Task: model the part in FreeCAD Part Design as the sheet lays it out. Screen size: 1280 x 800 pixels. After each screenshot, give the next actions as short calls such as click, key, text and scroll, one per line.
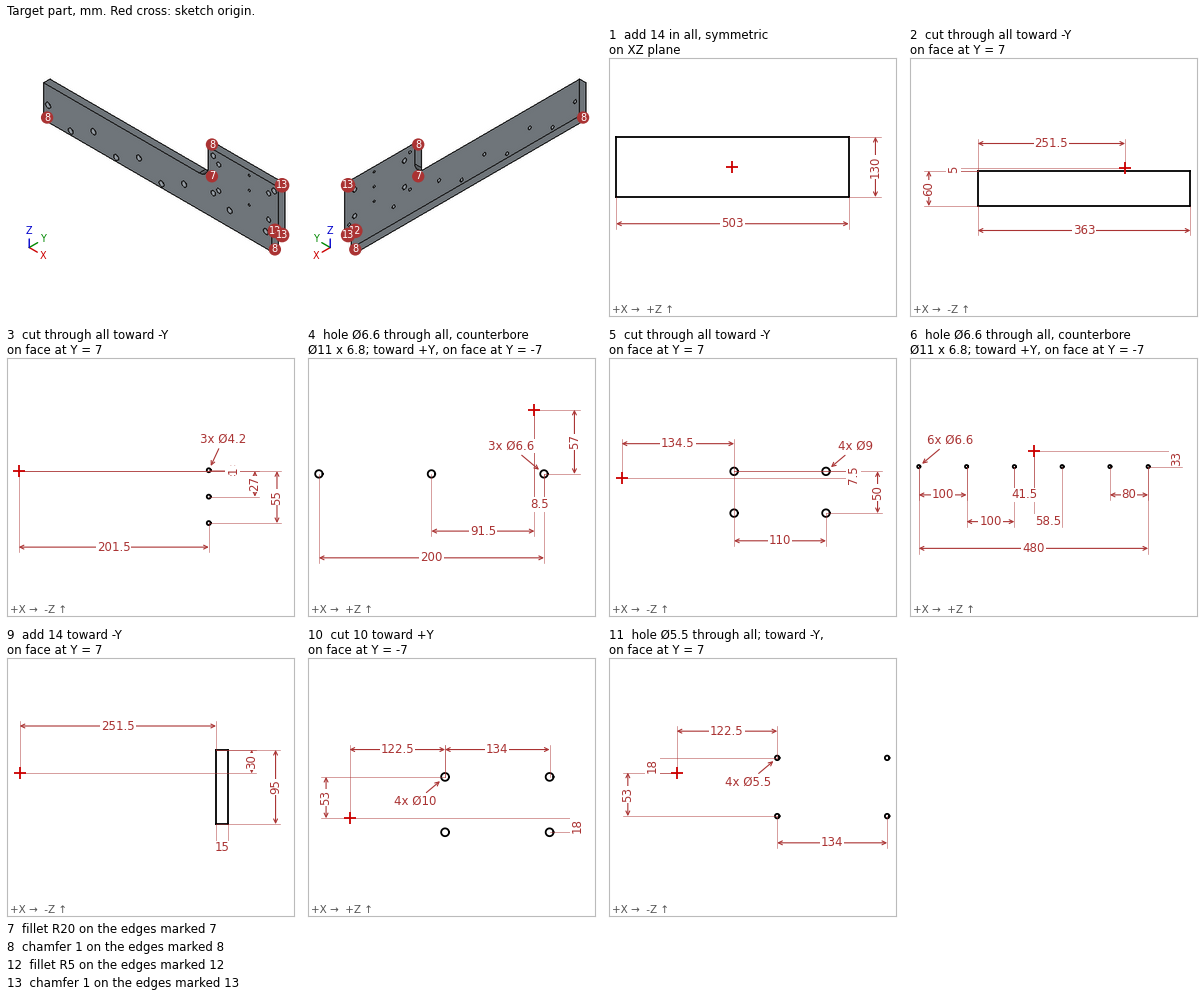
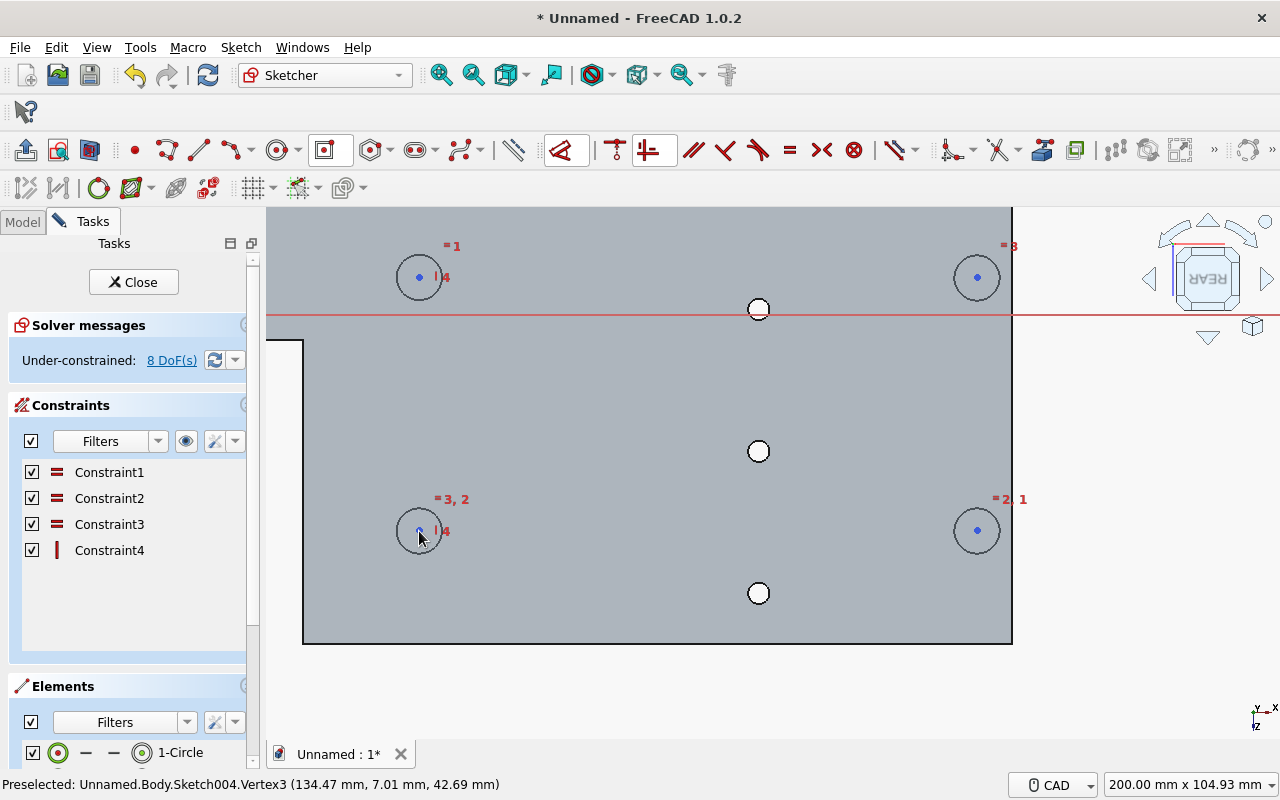
click(977, 531)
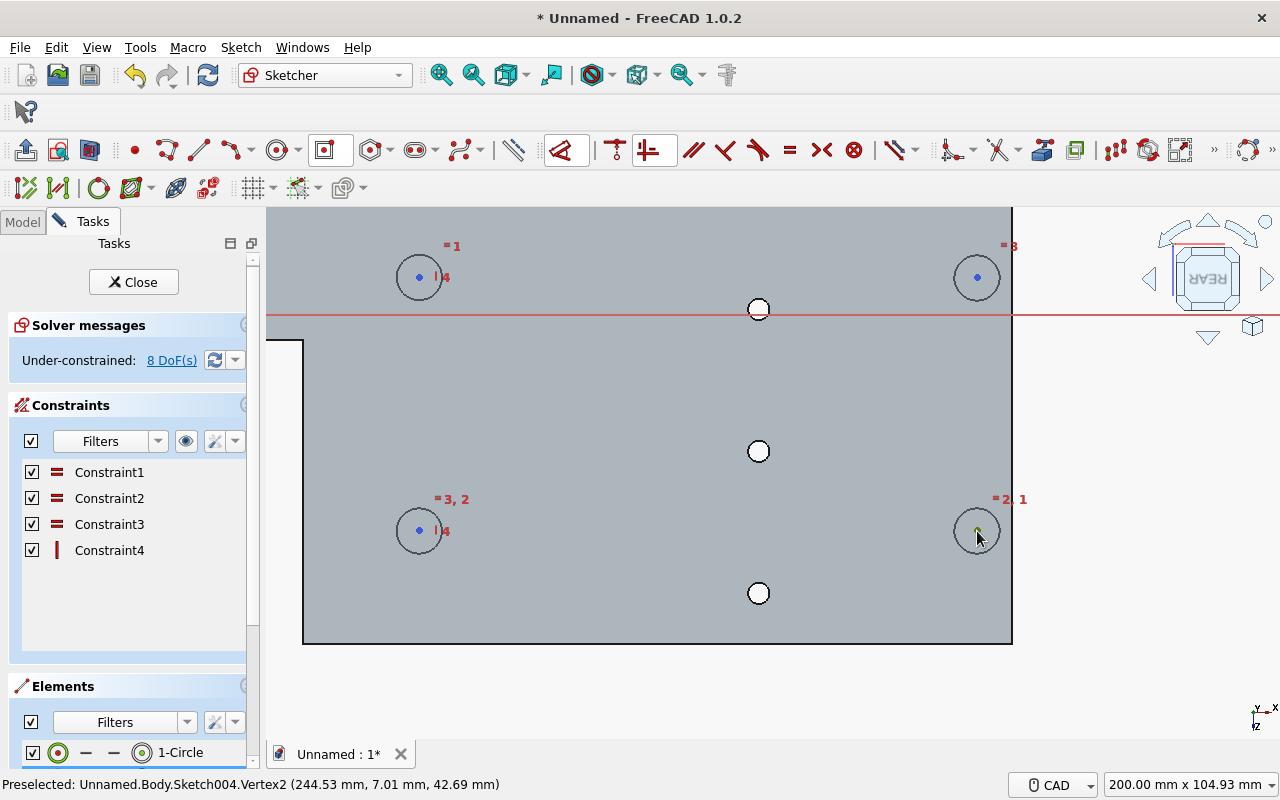
click(419, 531)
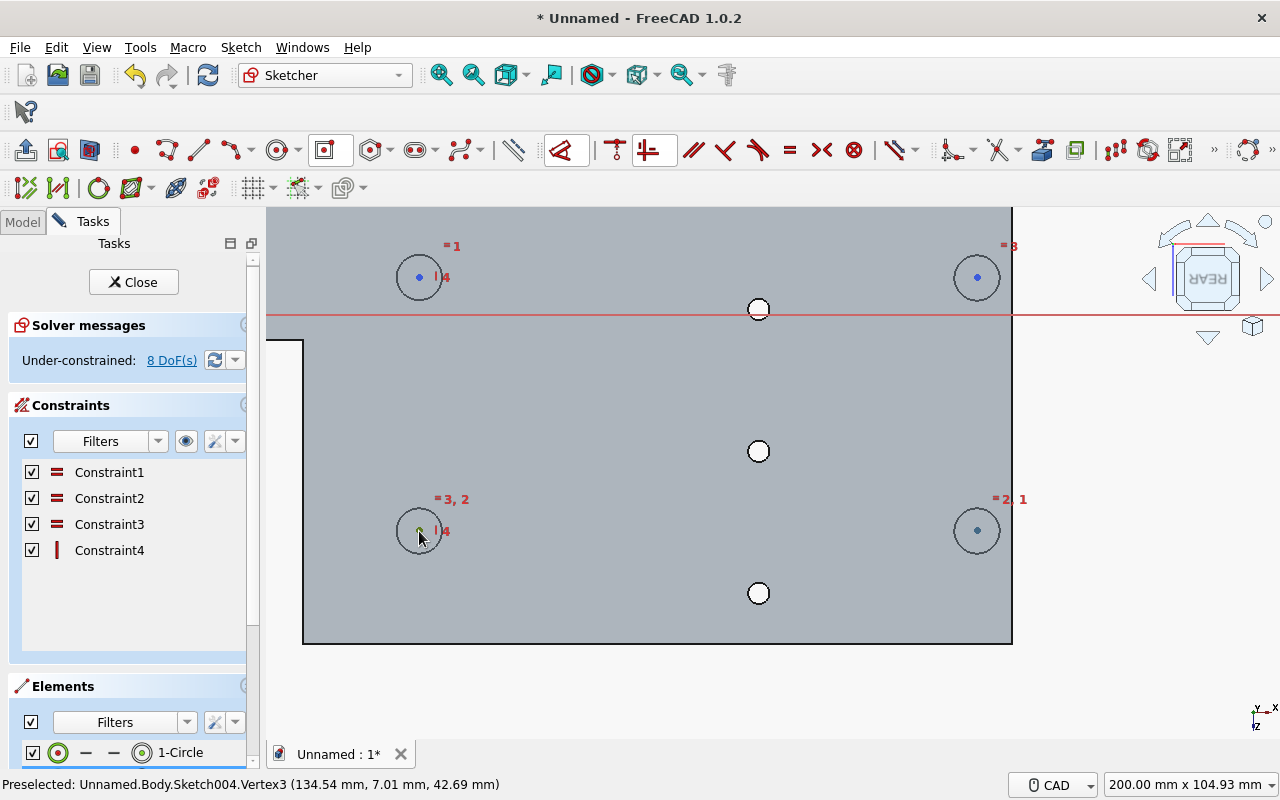
key(h)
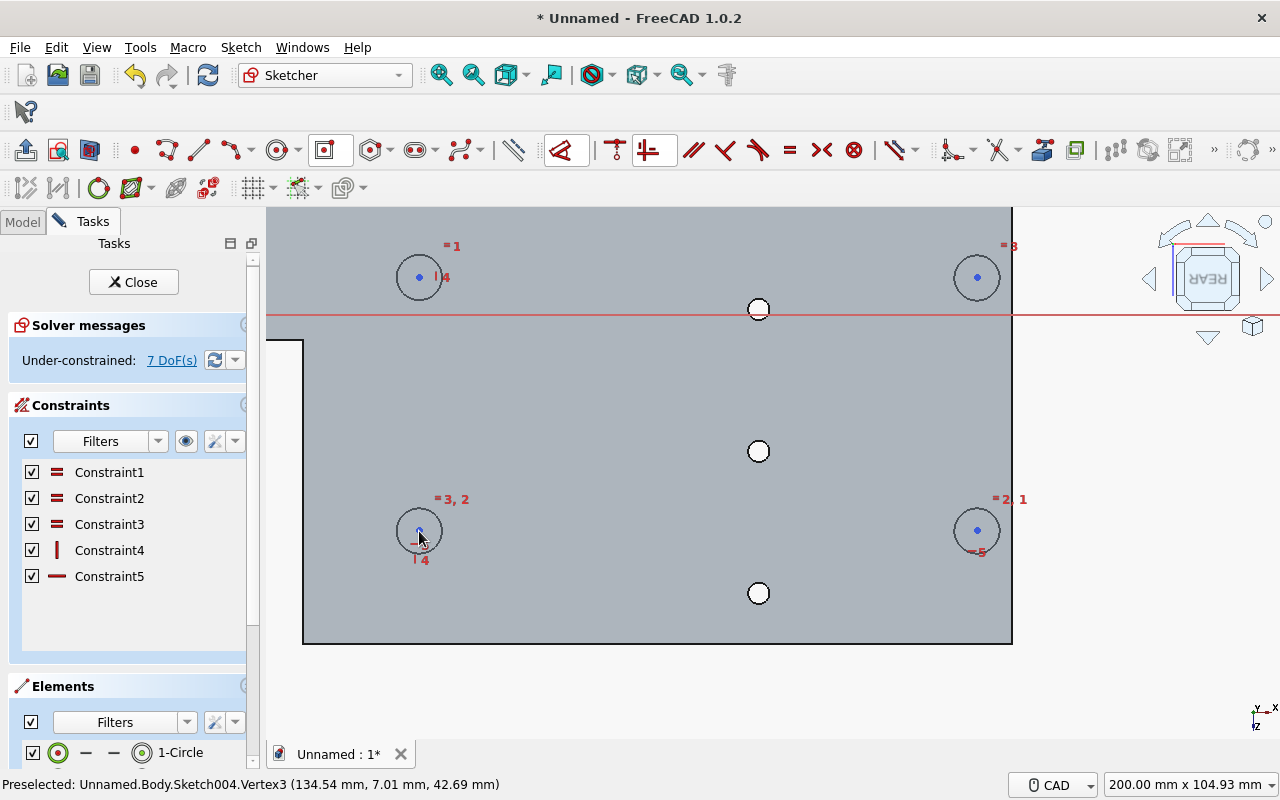
click(977, 531)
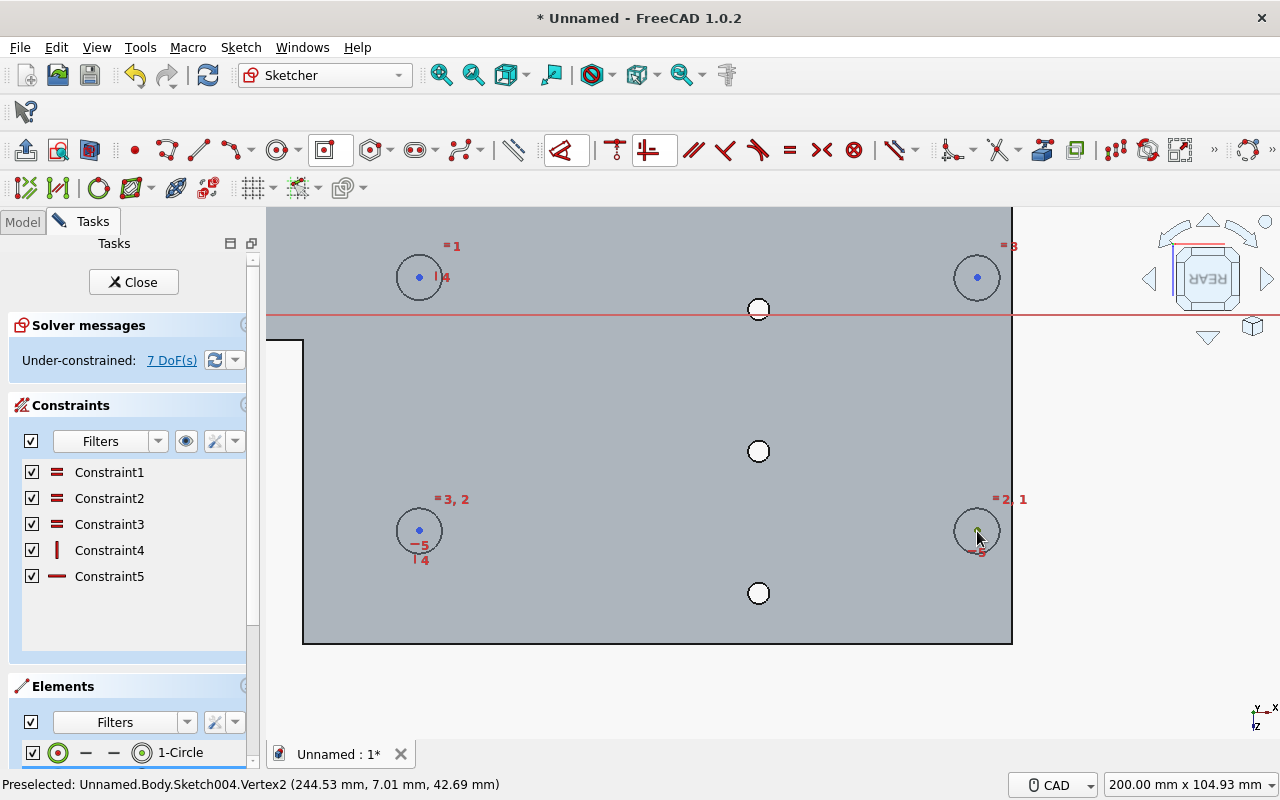
click(977, 278)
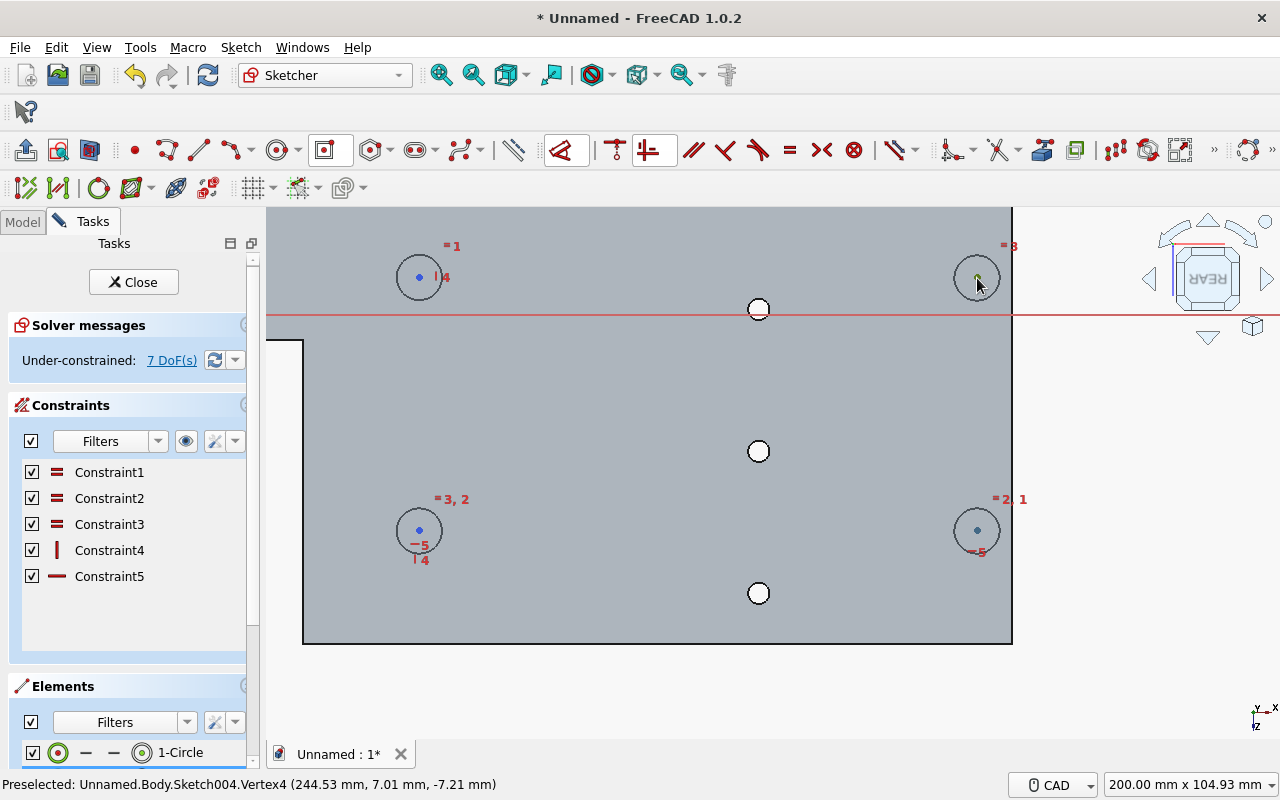
key(v)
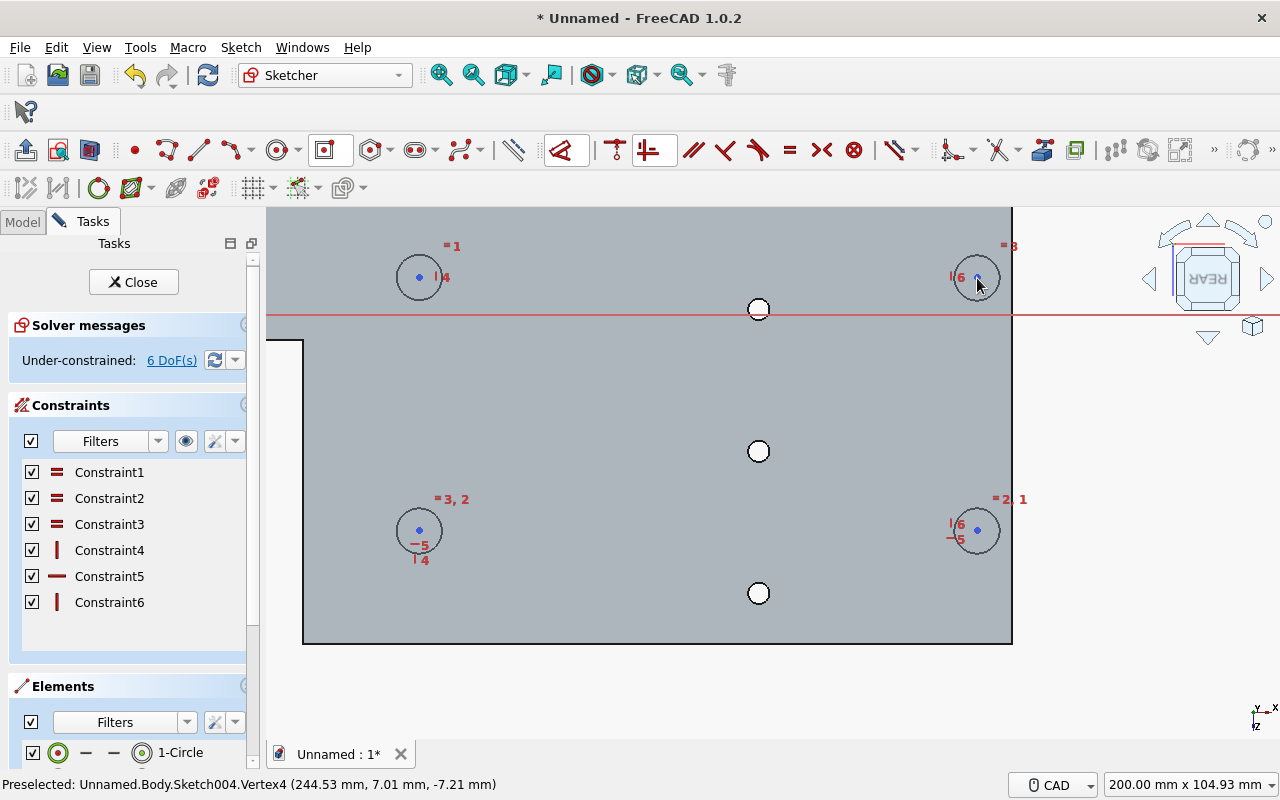
click(419, 277)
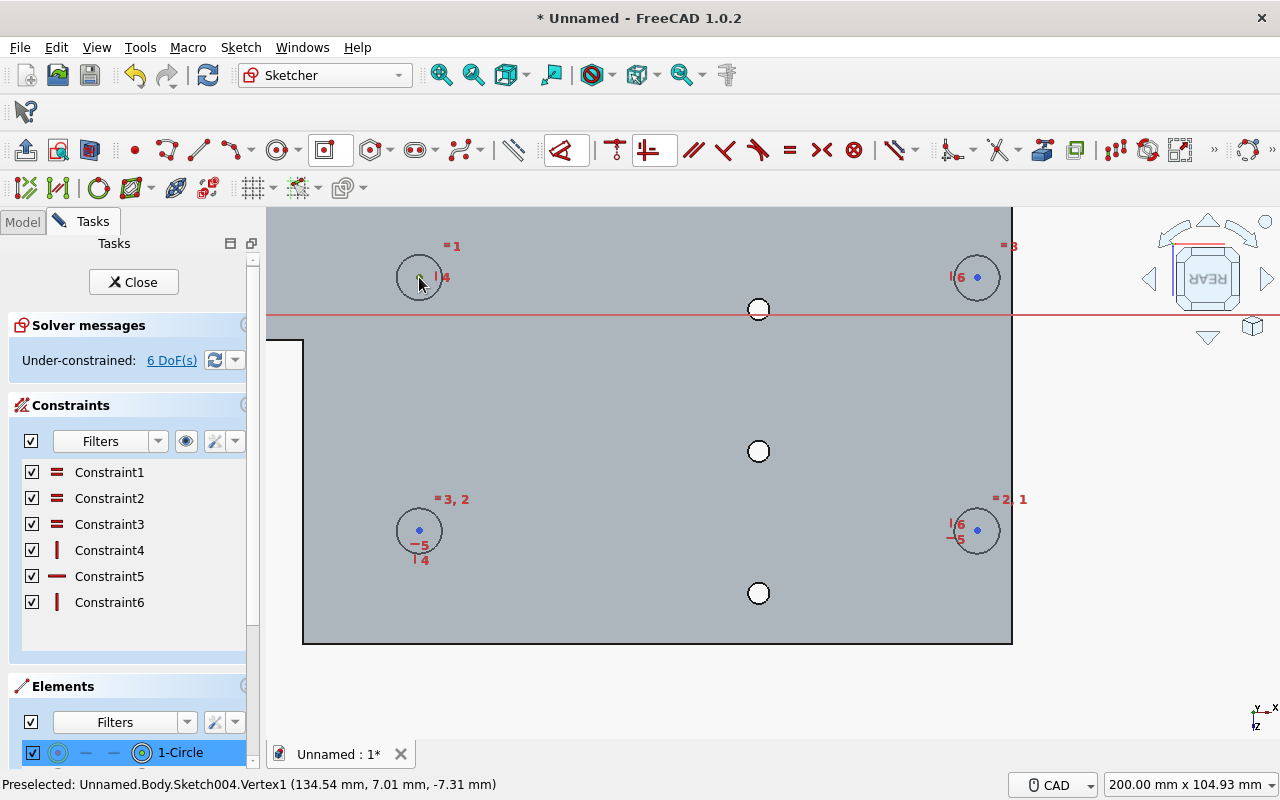
click(977, 278)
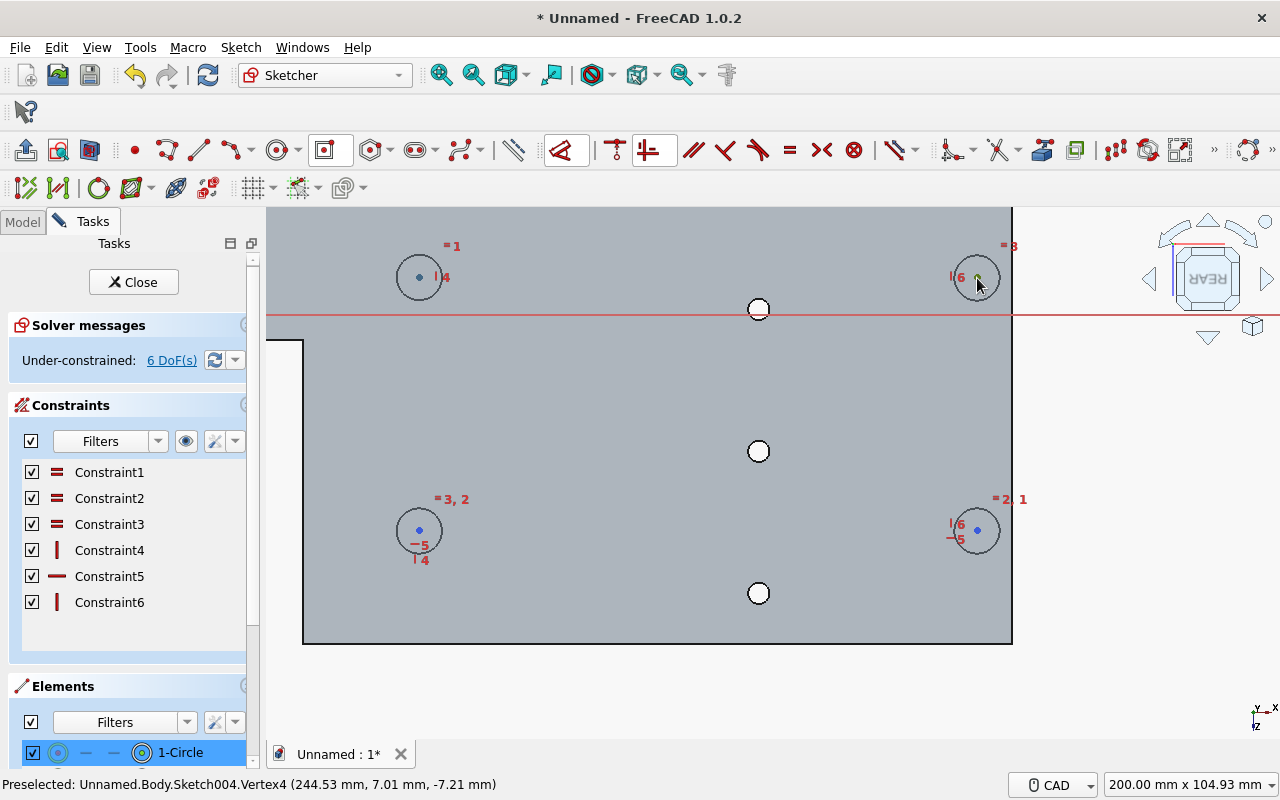
key(h)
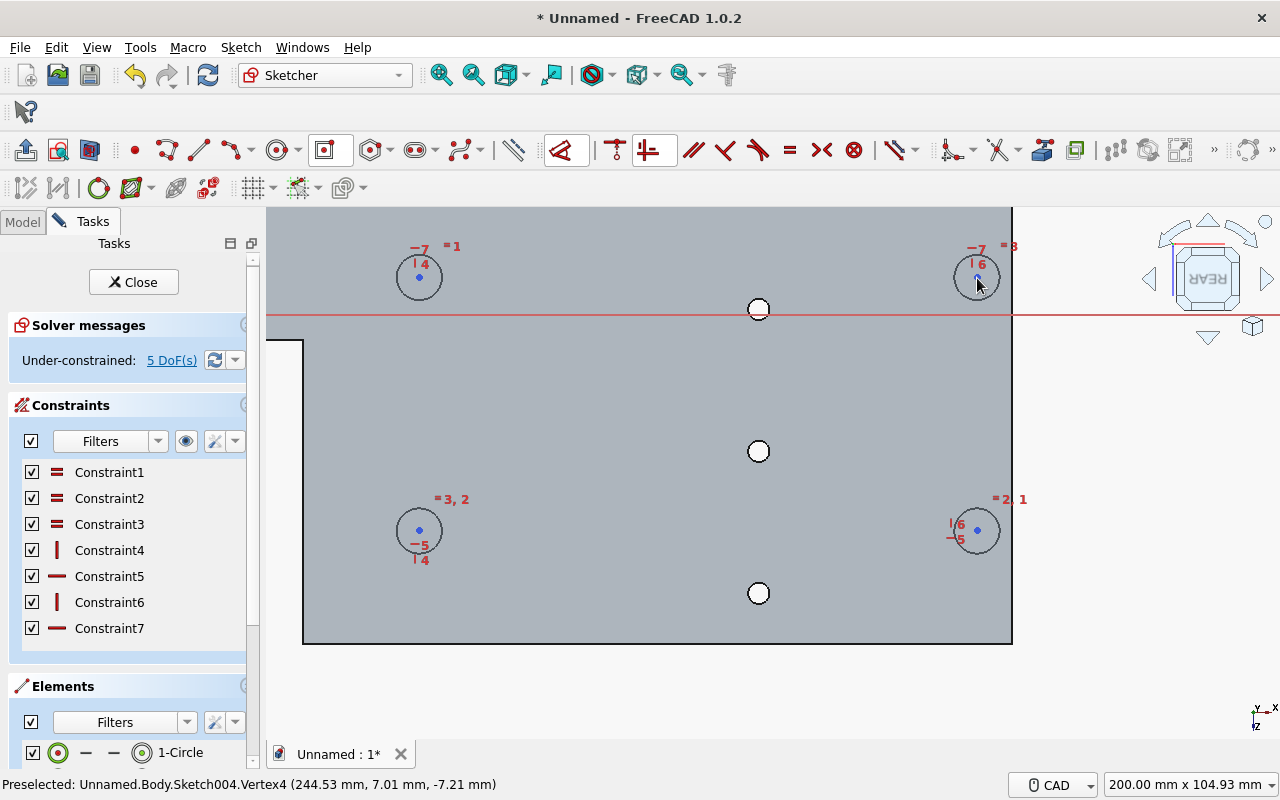
click(435, 261)